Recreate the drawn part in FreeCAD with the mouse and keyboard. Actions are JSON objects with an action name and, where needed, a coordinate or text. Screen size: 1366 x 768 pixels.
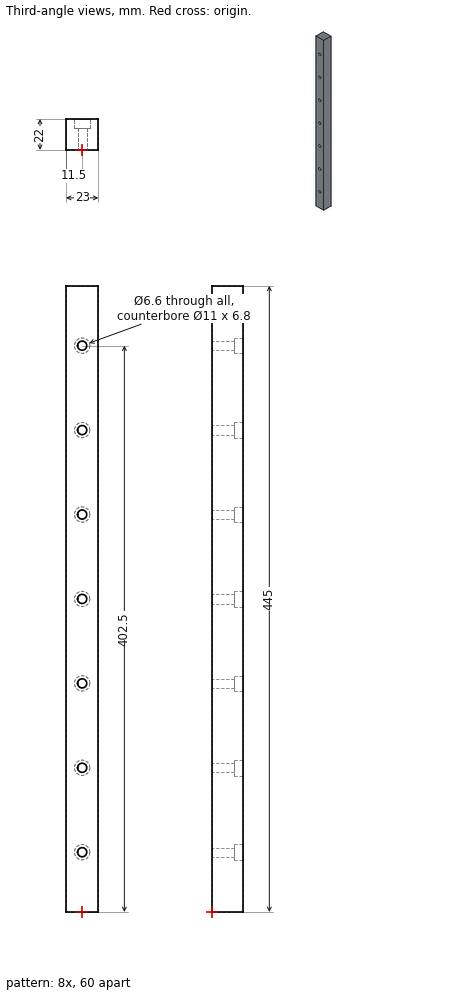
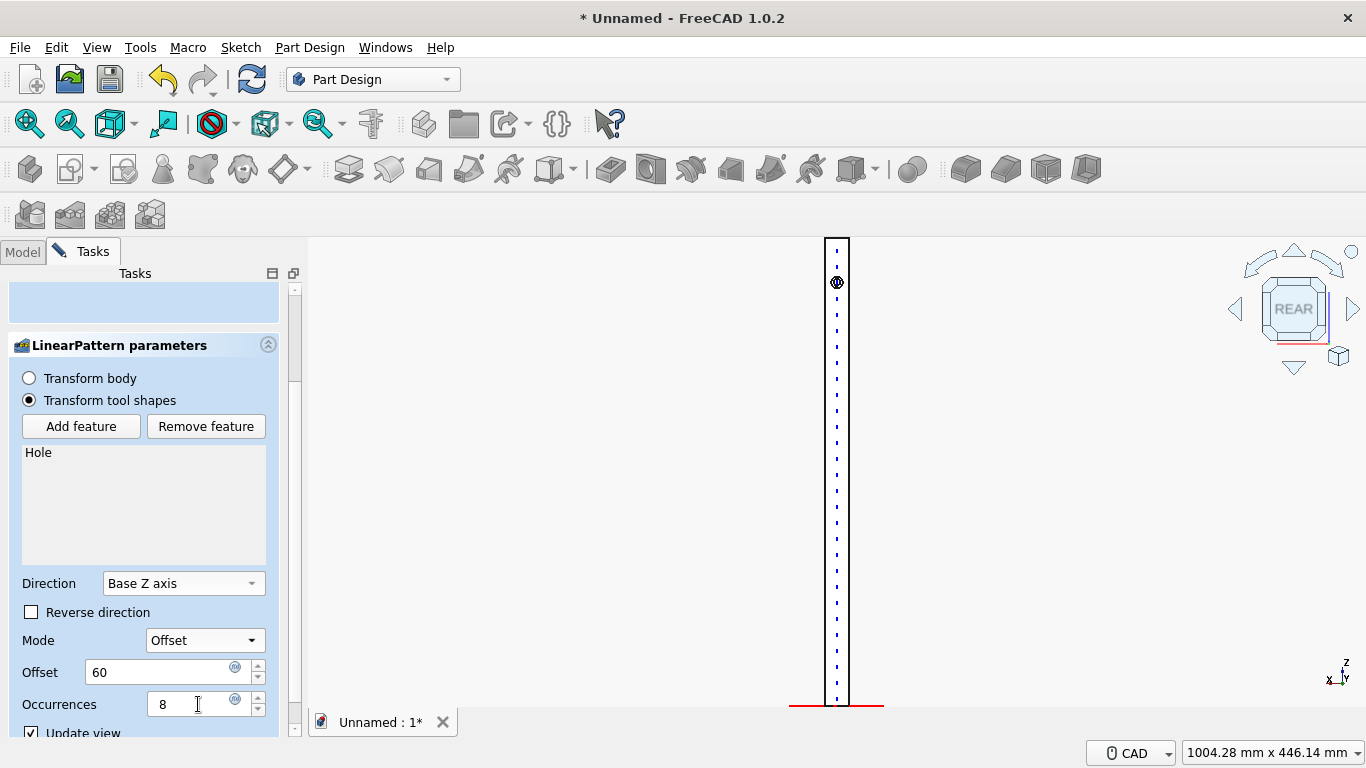
{"action": "left_click", "coordinate": [30, 612]}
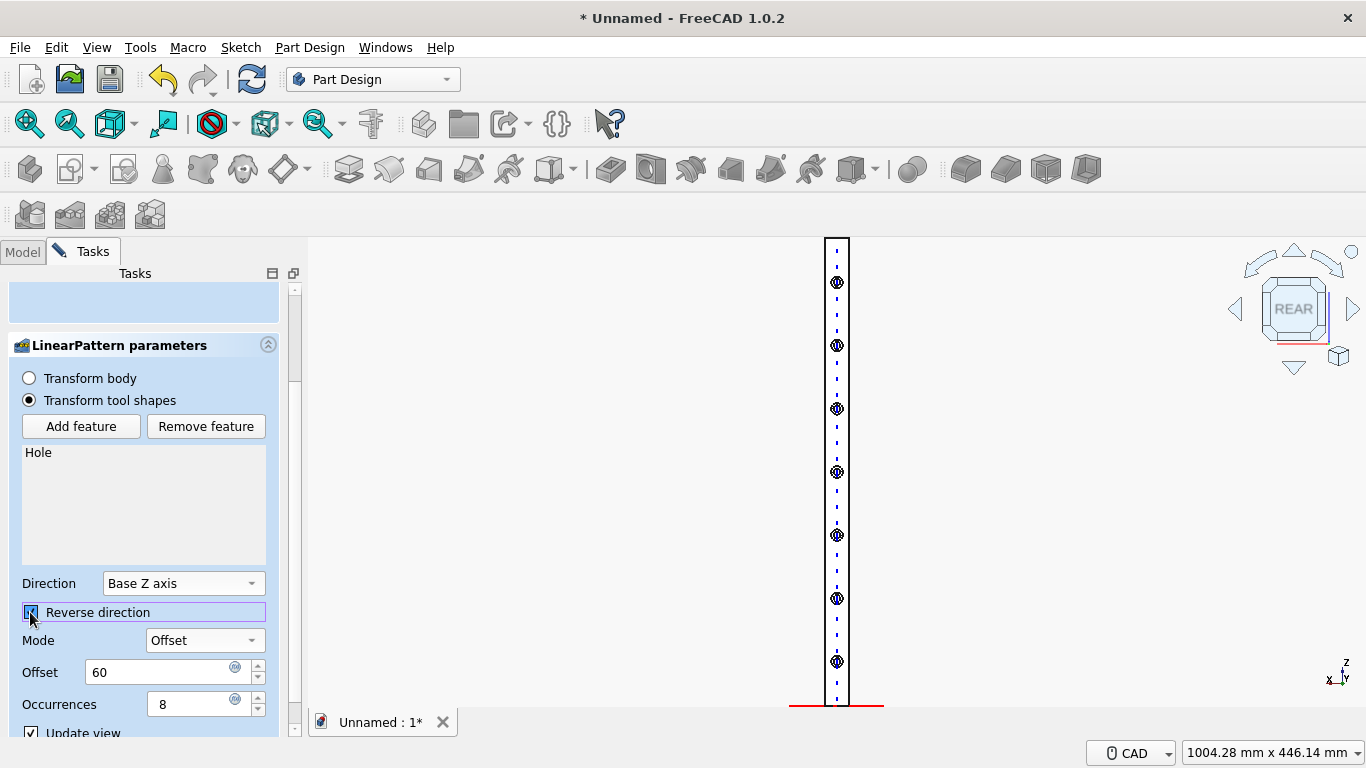
{"action": "scroll", "coordinate": [295, 510], "scroll_direction": "up", "scroll_amount": 3}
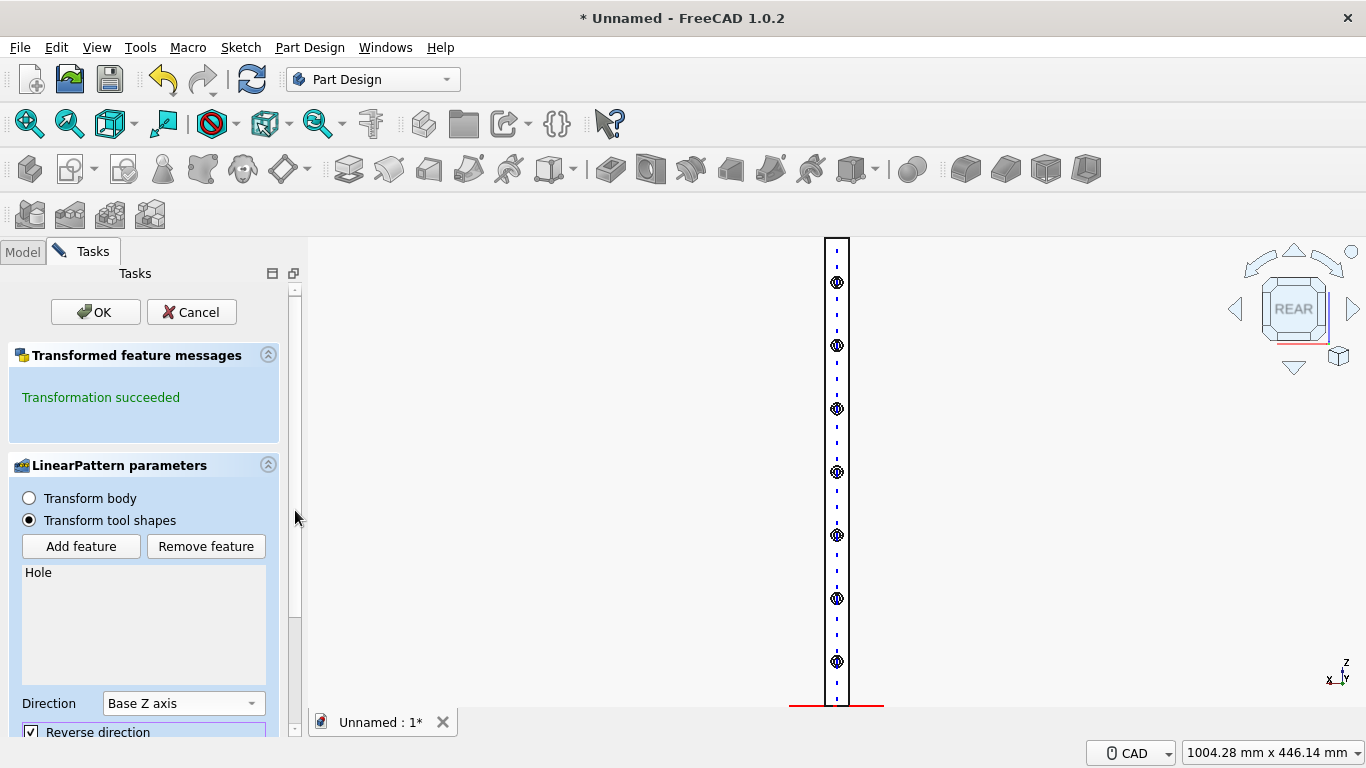
{"action": "left_click", "coordinate": [96, 312]}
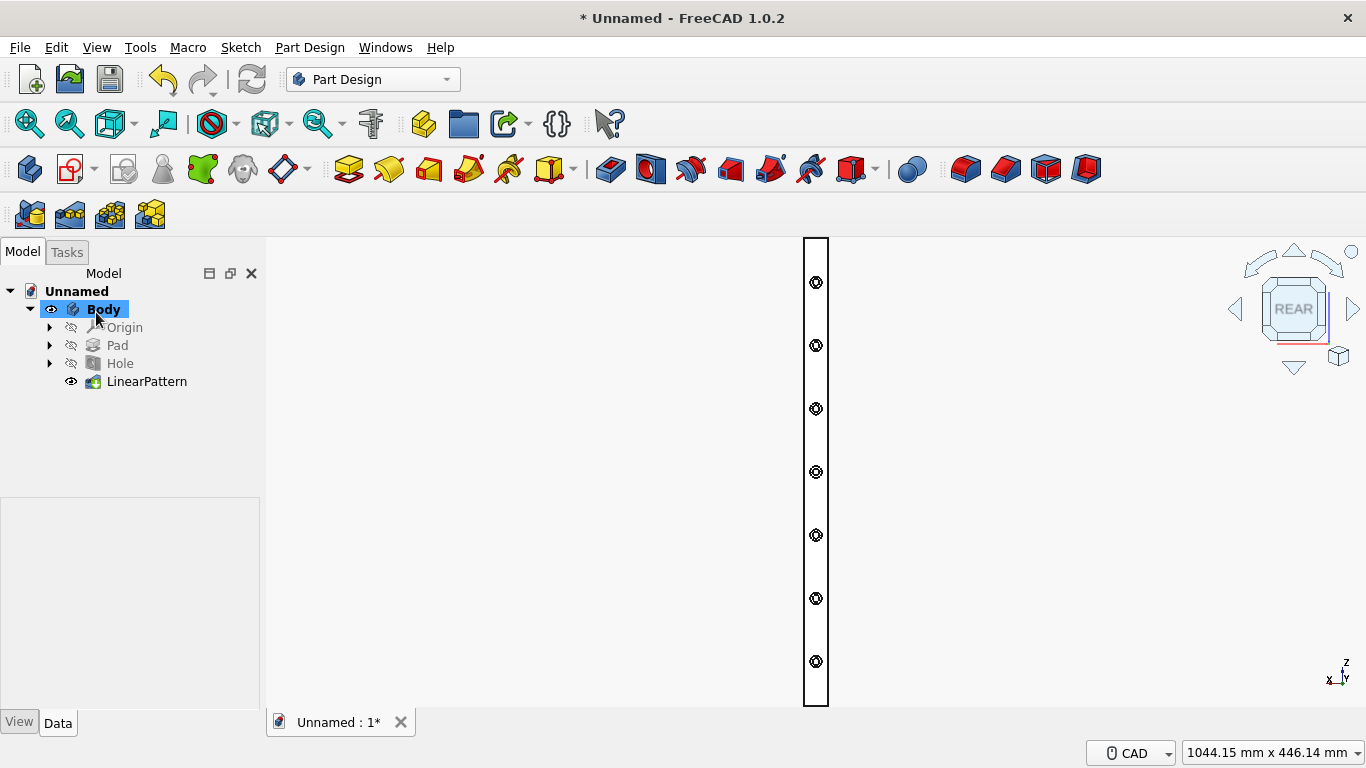
{"action": "key", "text": "0"}